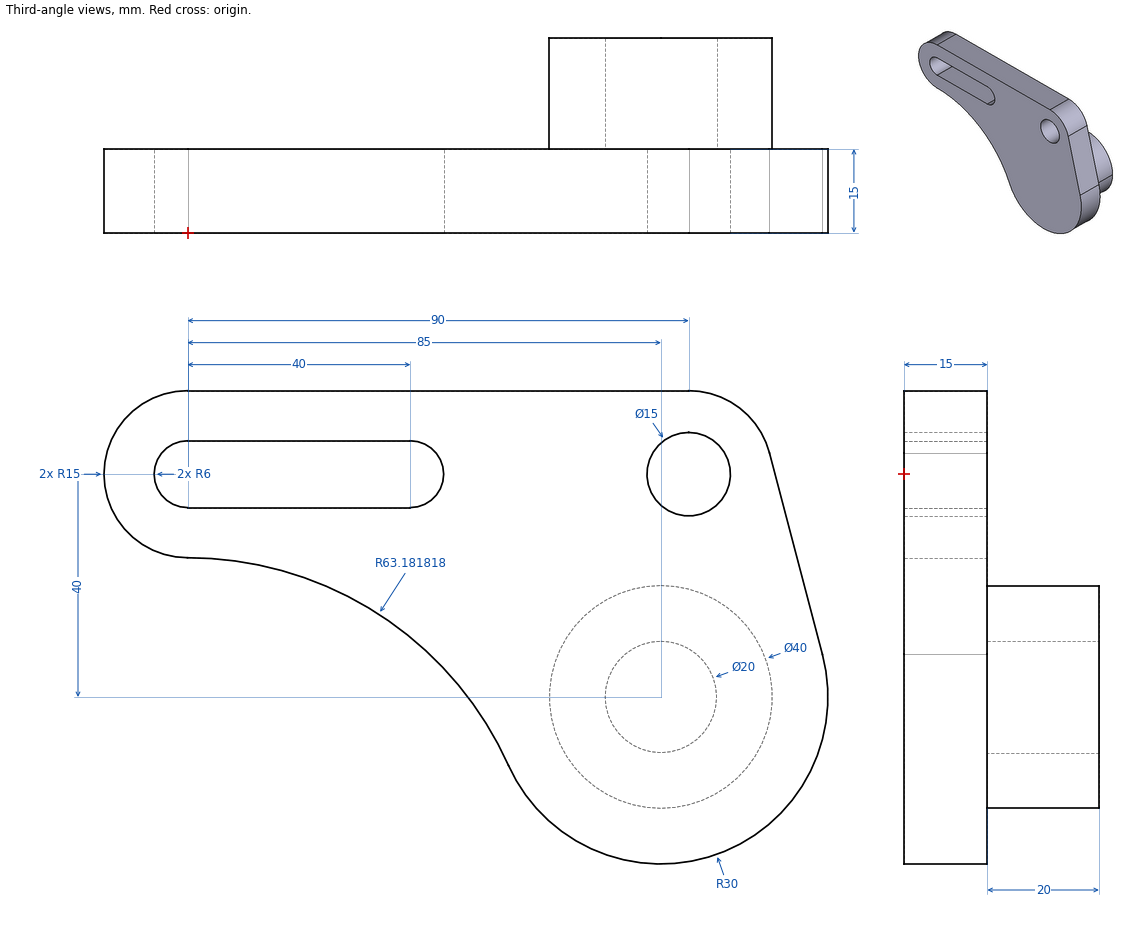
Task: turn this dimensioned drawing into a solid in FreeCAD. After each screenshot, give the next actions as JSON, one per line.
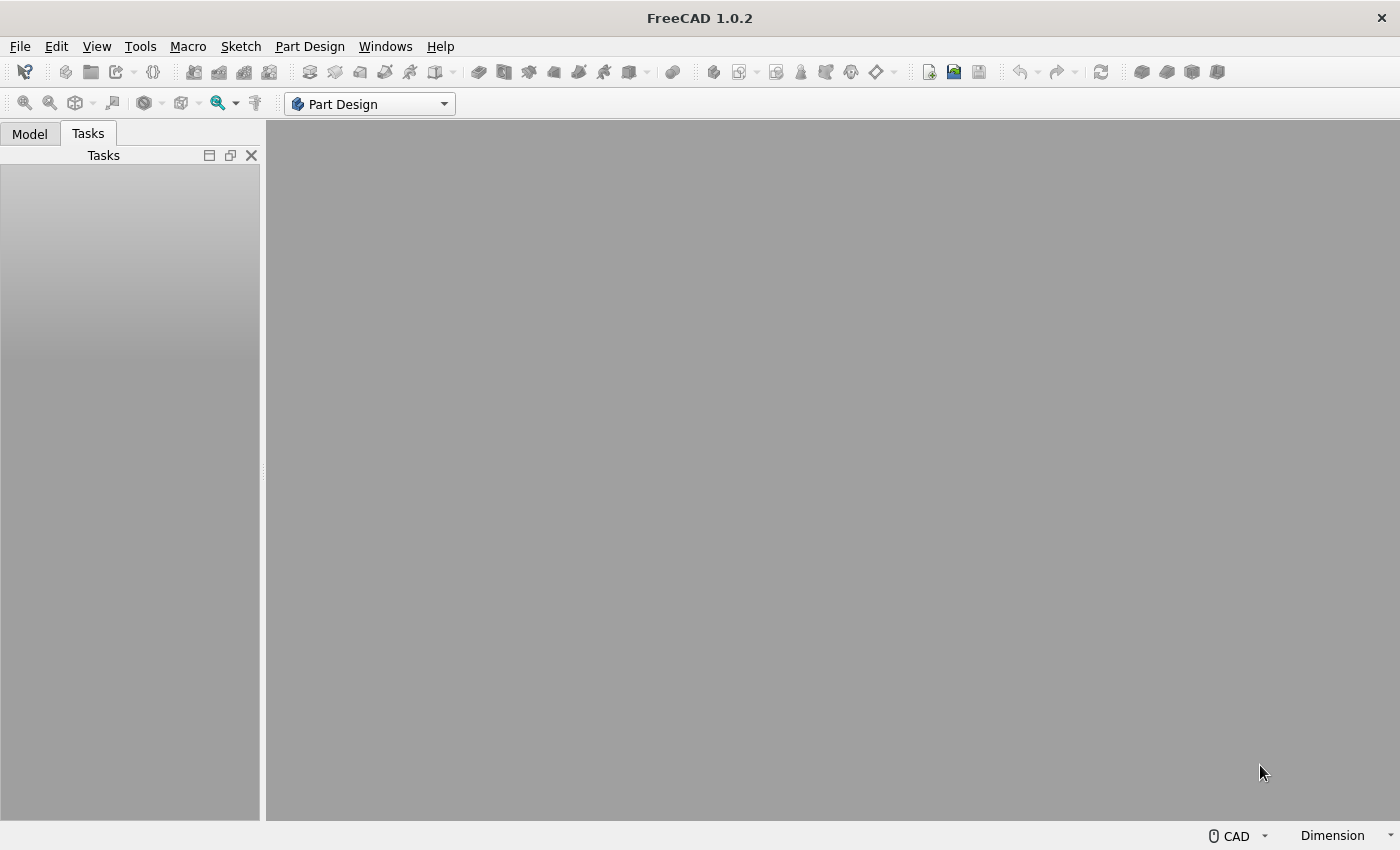
{"action": "left_click", "coordinate": [929, 72]}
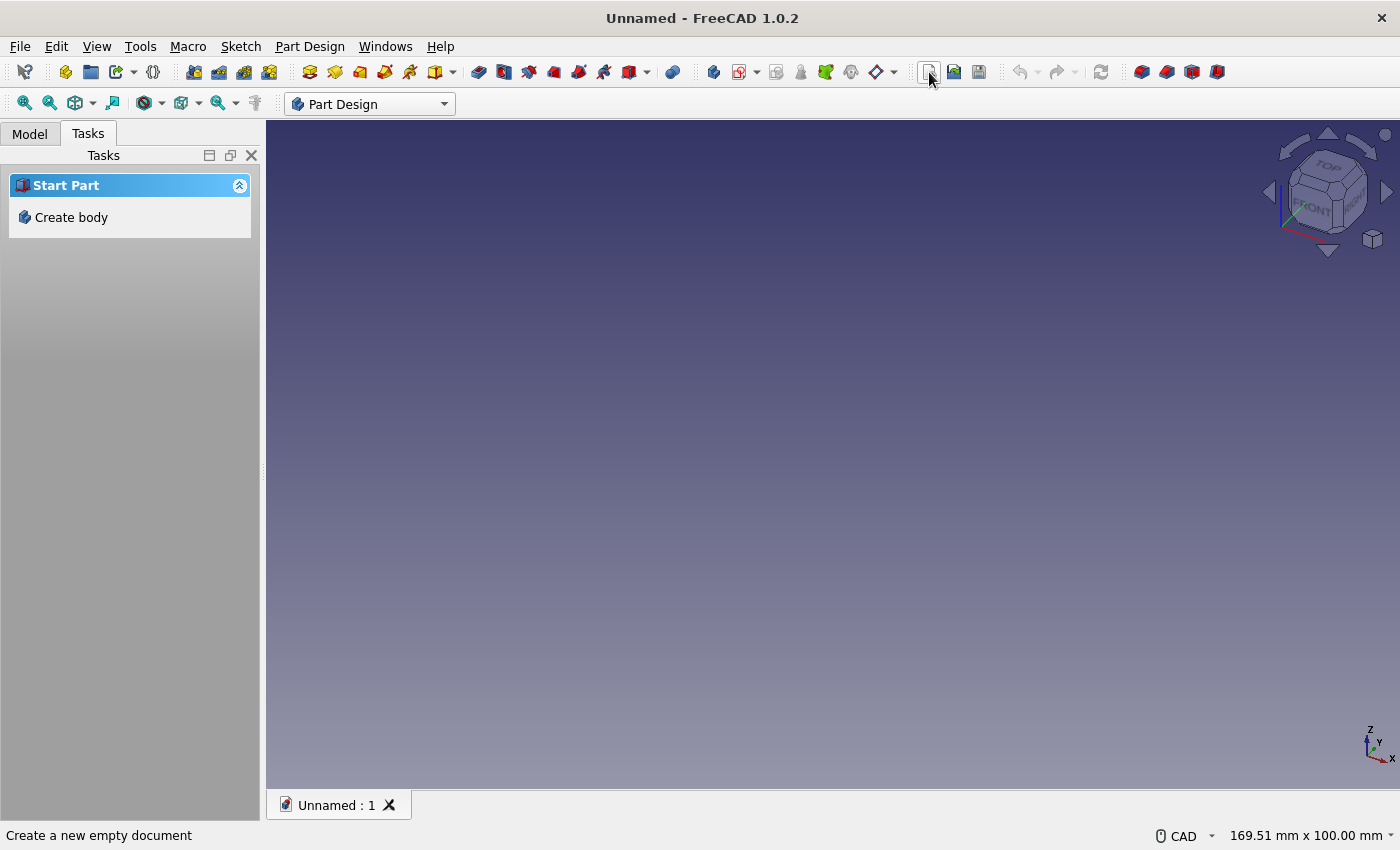
{"action": "left_click", "coordinate": [738, 72]}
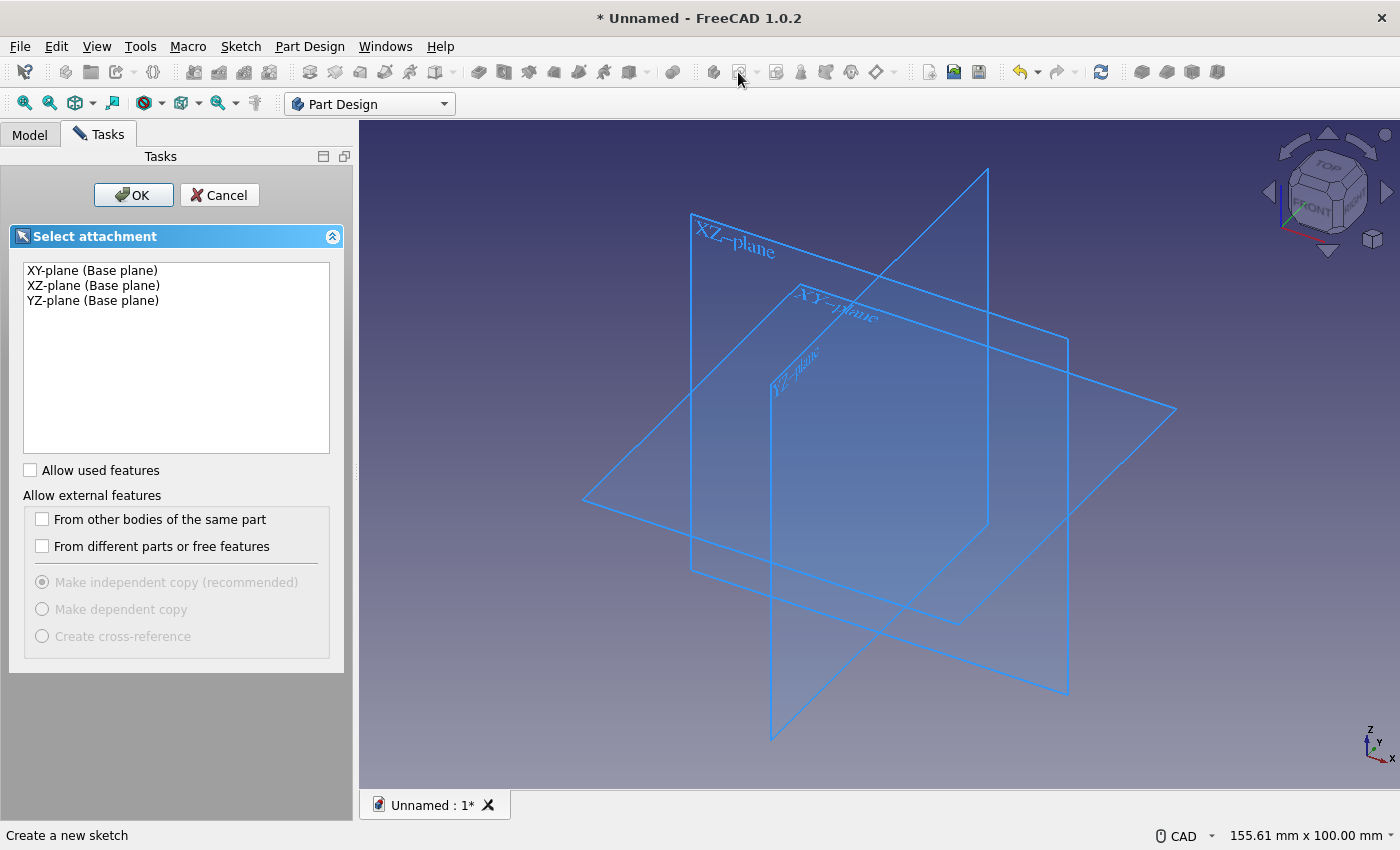
{"action": "left_click", "coordinate": [84, 286]}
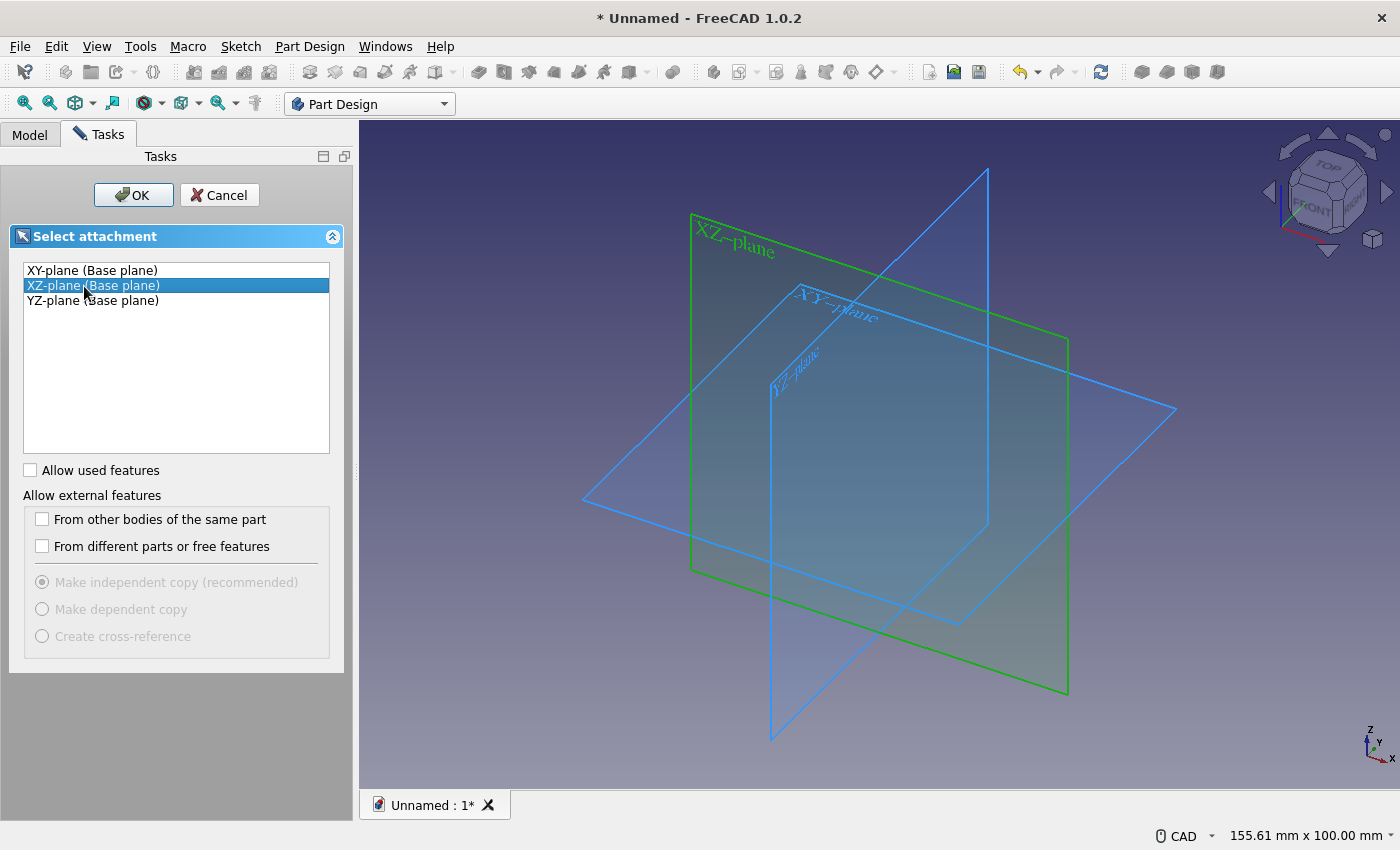
{"action": "left_click", "coordinate": [134, 195]}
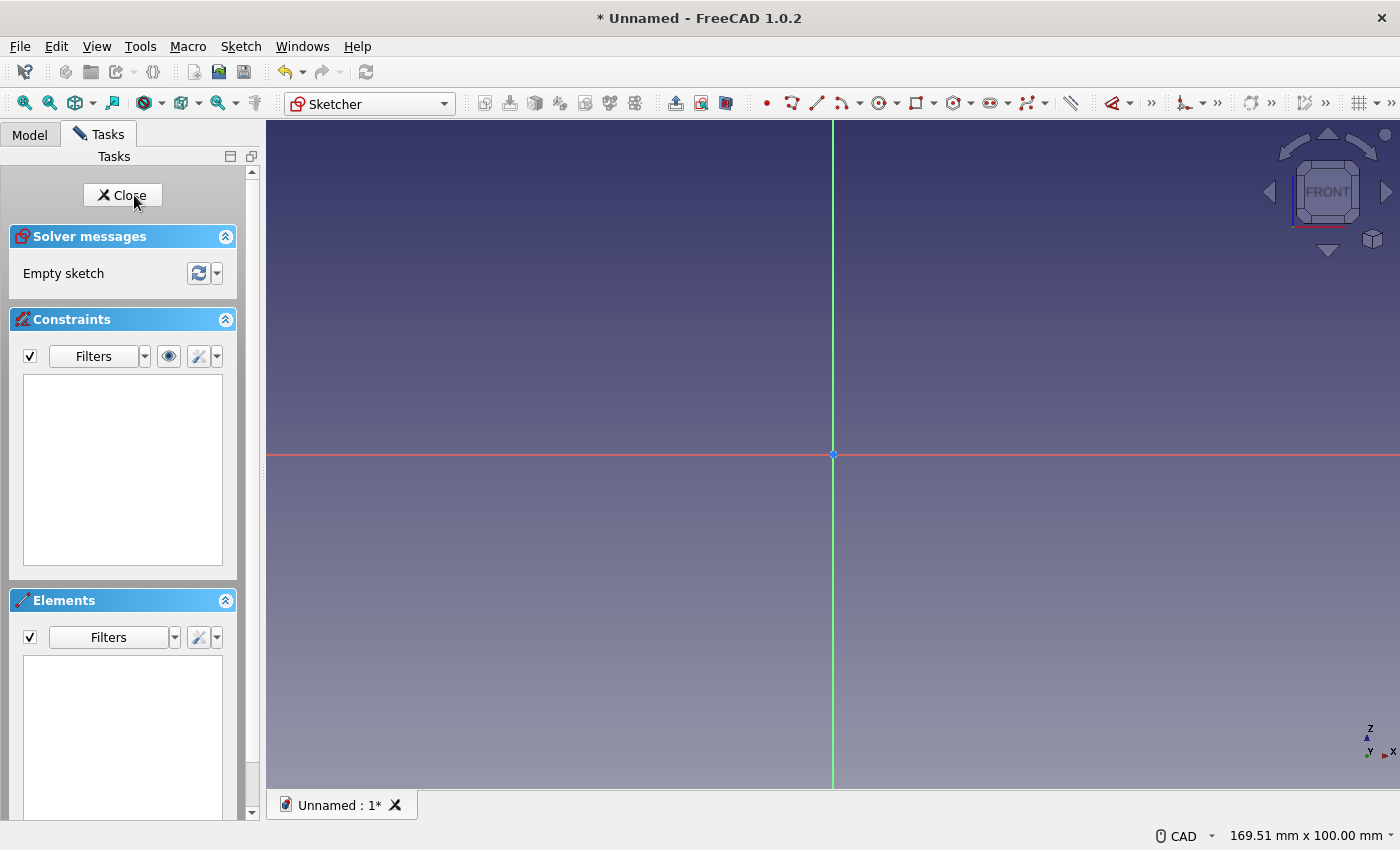
{"action": "scroll", "coordinate": [294, 148], "scroll_direction": "down", "scroll_amount": 2}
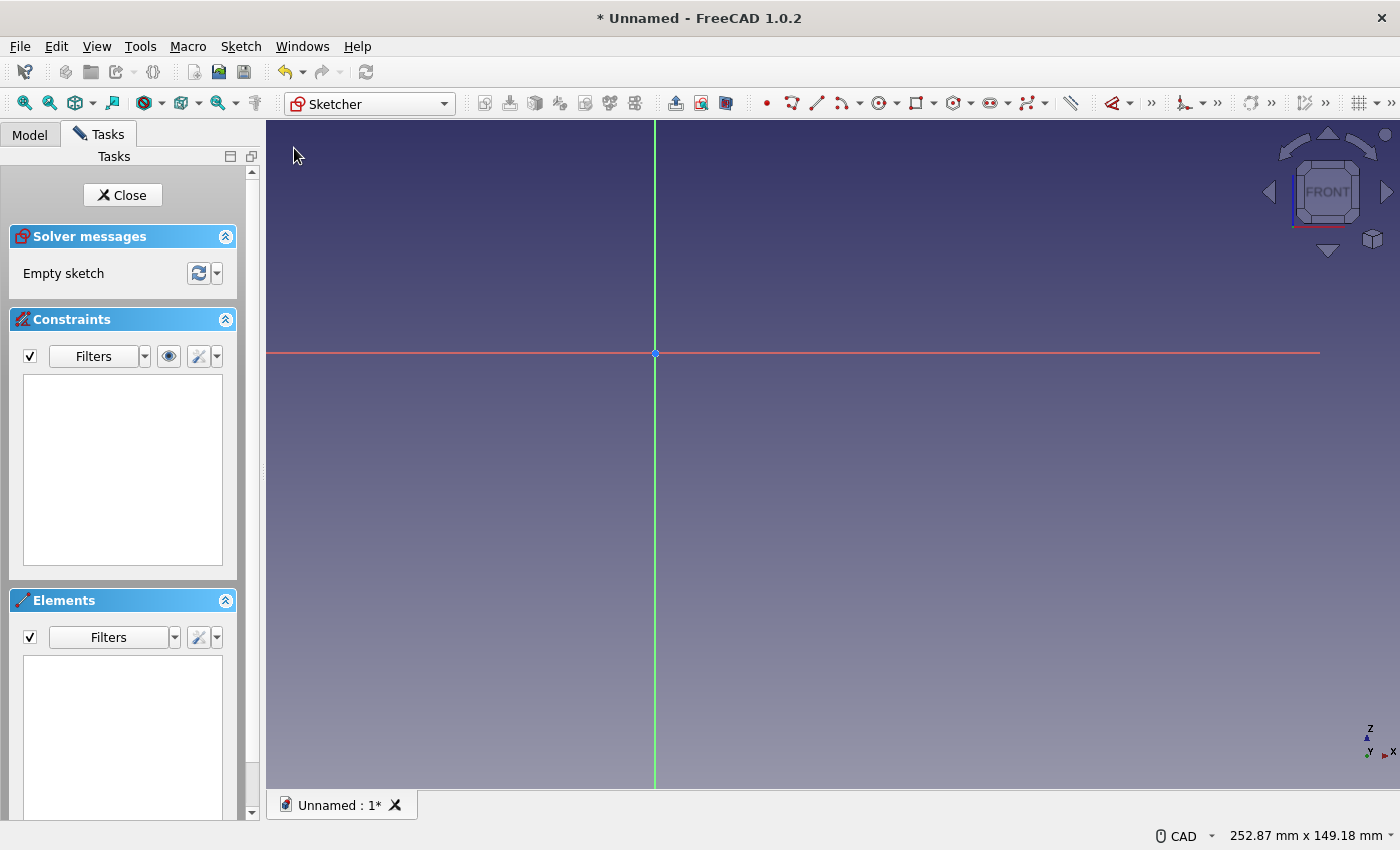
{"action": "left_click", "coordinate": [817, 104]}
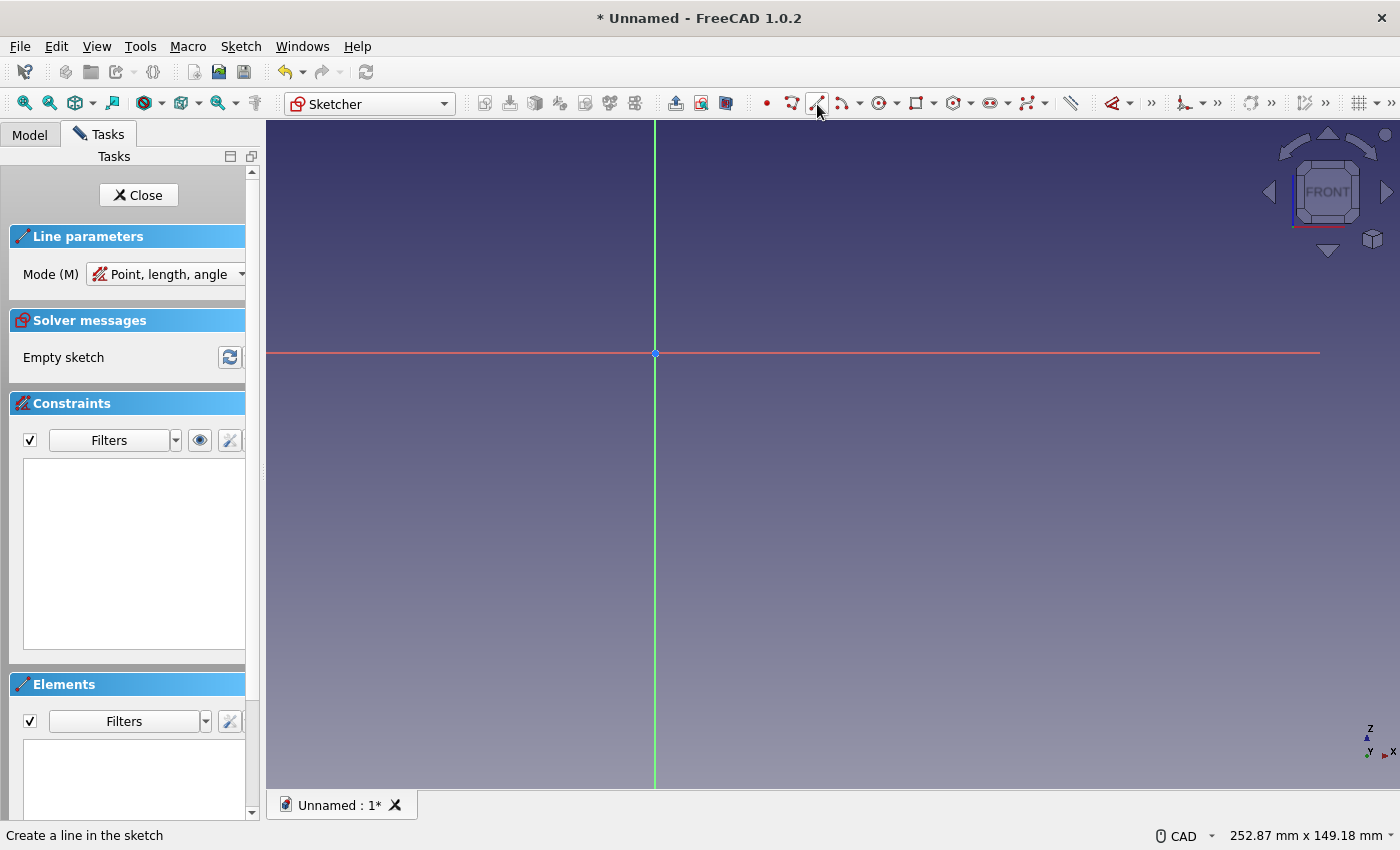
{"action": "left_click", "coordinate": [1124, 336]}
{"action": "left_click", "coordinate": [1167, 499]}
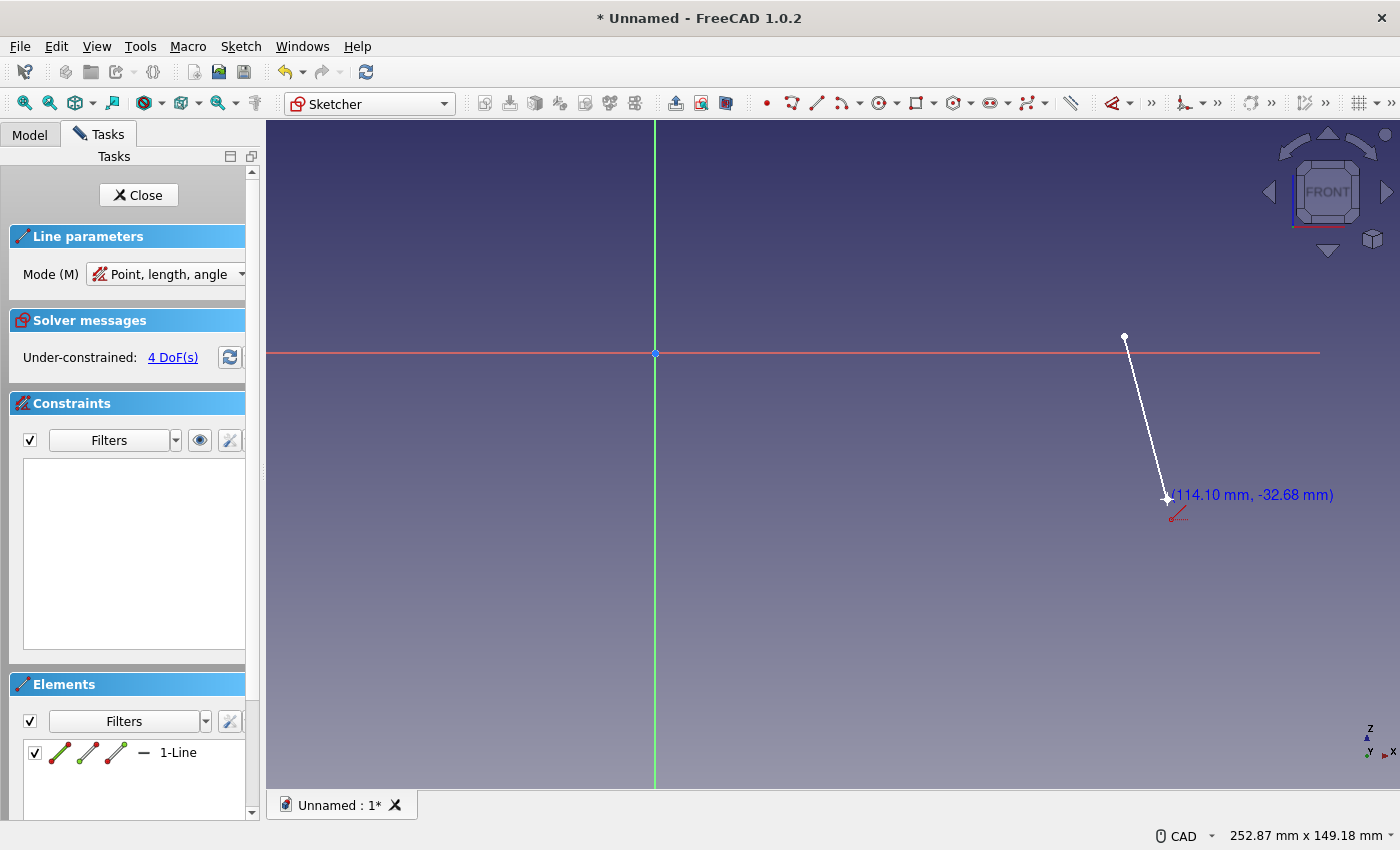
{"action": "left_click", "coordinate": [655, 286]}
{"action": "left_click", "coordinate": [1059, 286]}